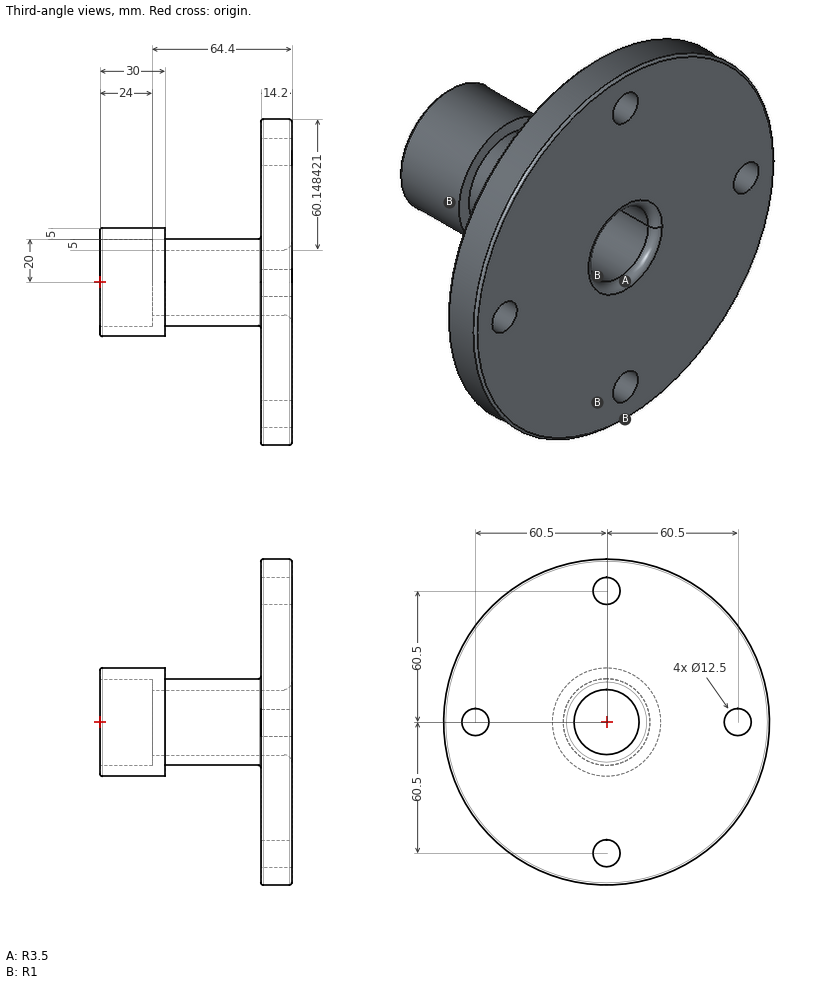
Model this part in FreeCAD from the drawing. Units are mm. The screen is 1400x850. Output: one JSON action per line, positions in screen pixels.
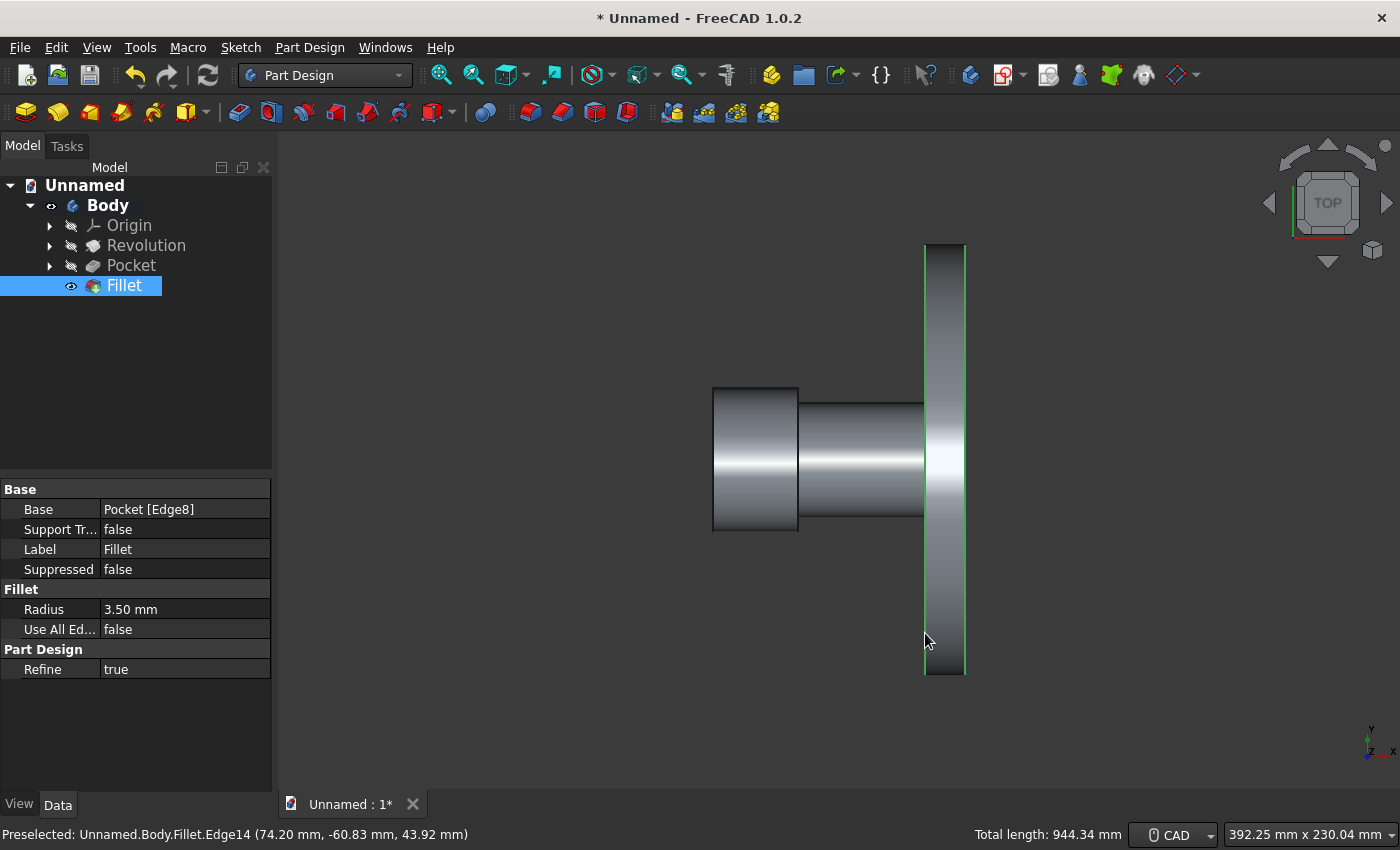
{"action": "left_click", "coordinate": [713, 517], "text": "ctrl"}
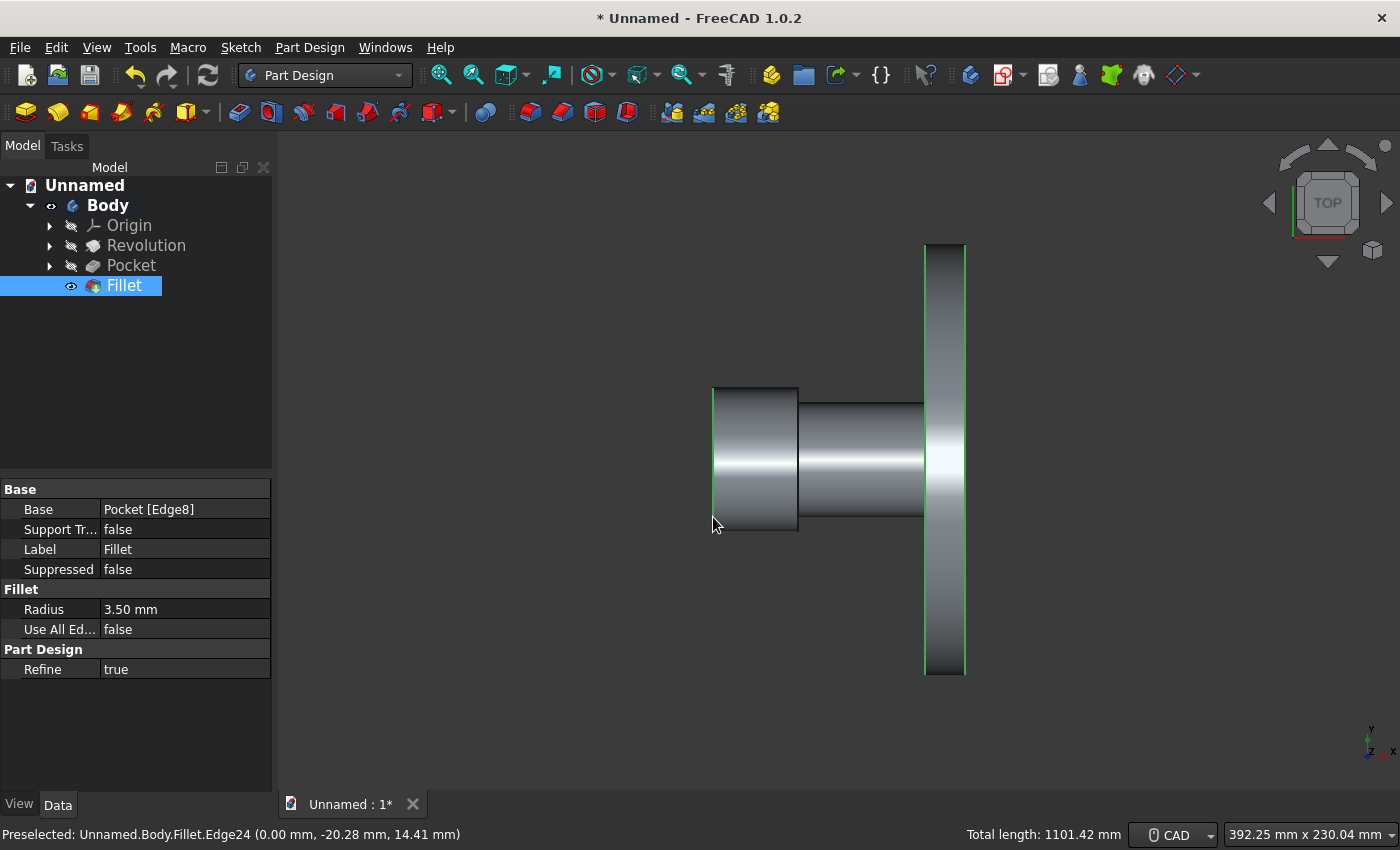
{"action": "key", "text": "0"}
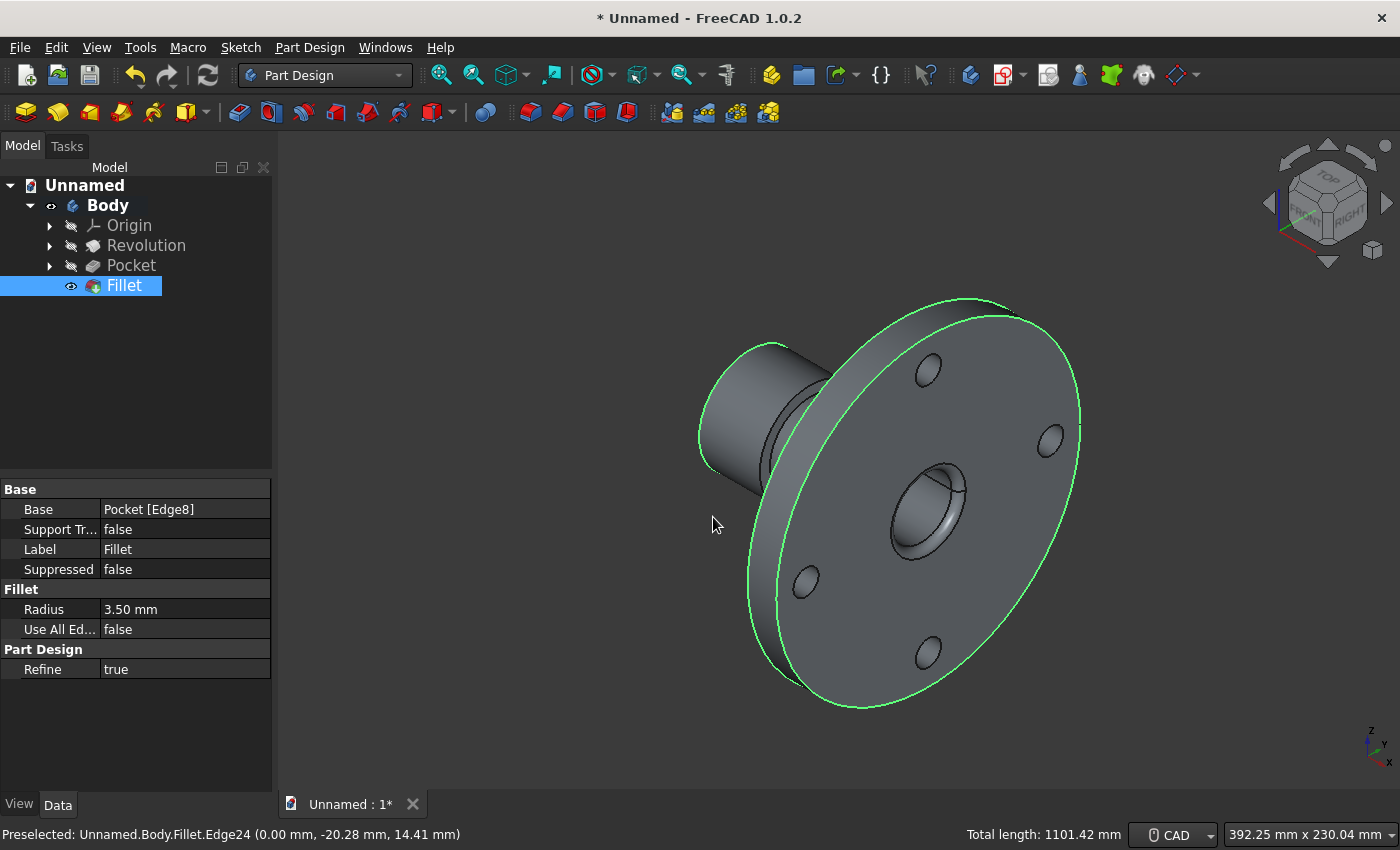
{"action": "key", "text": "1"}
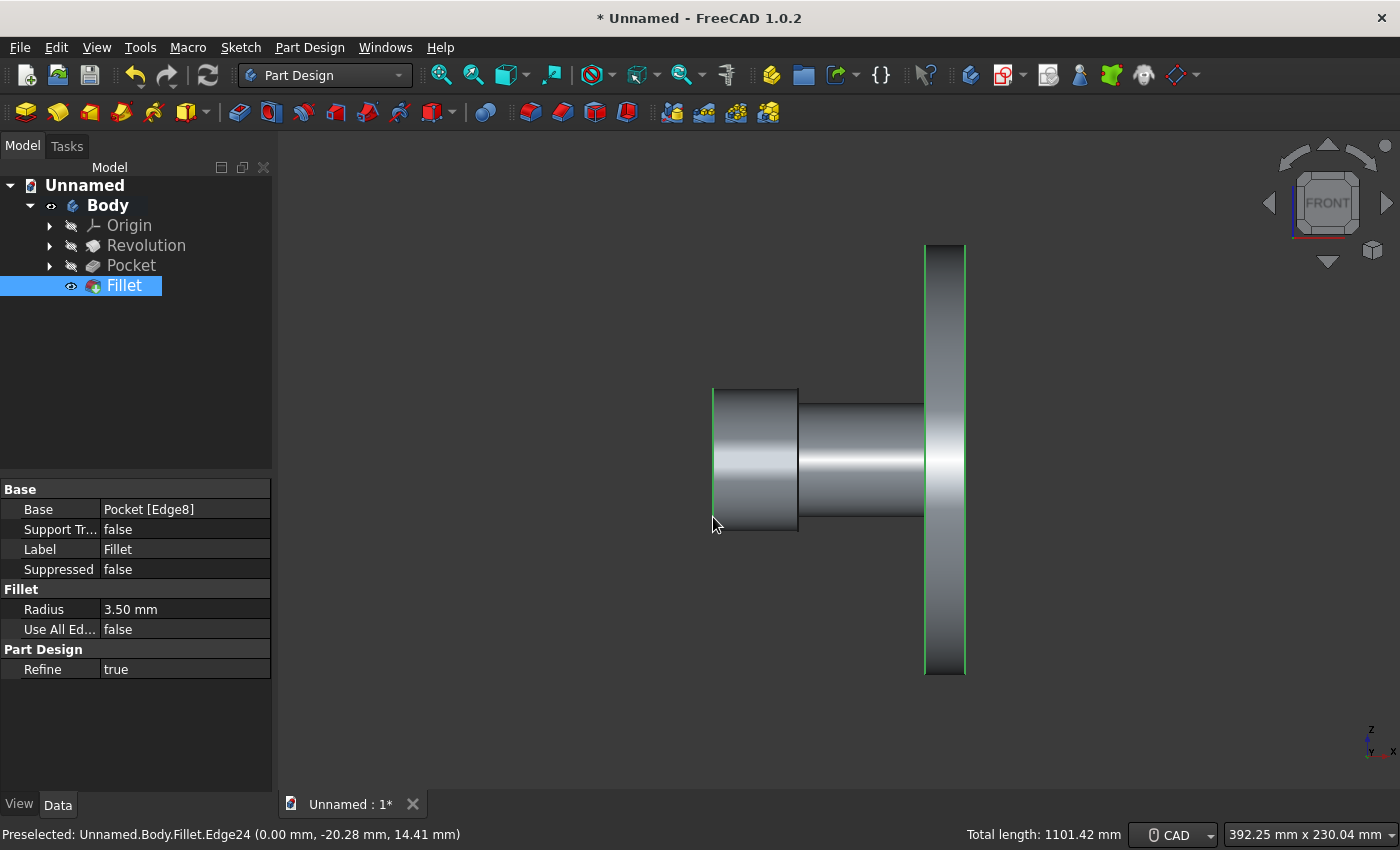
{"action": "key", "text": "3"}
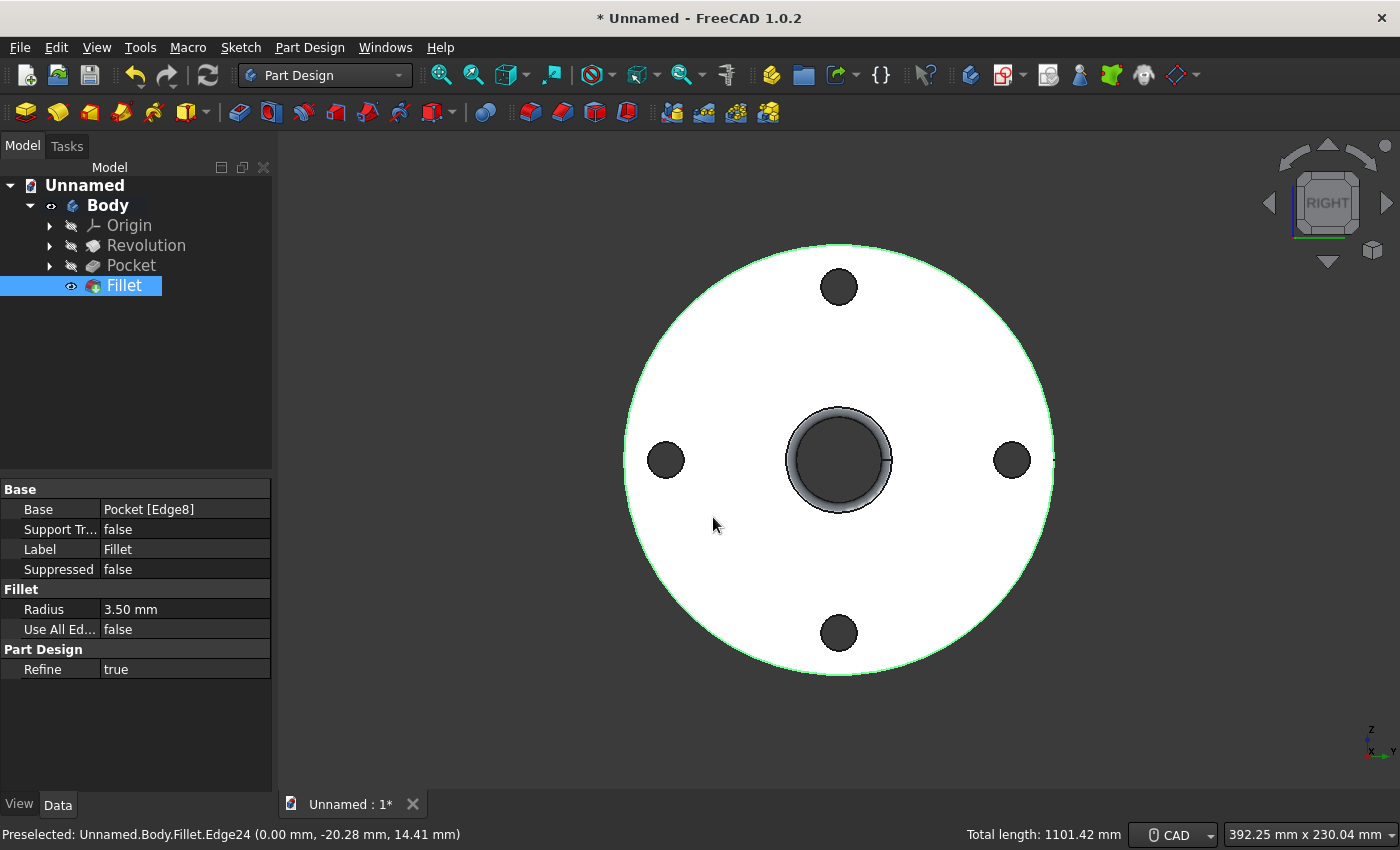
{"action": "key", "text": "5"}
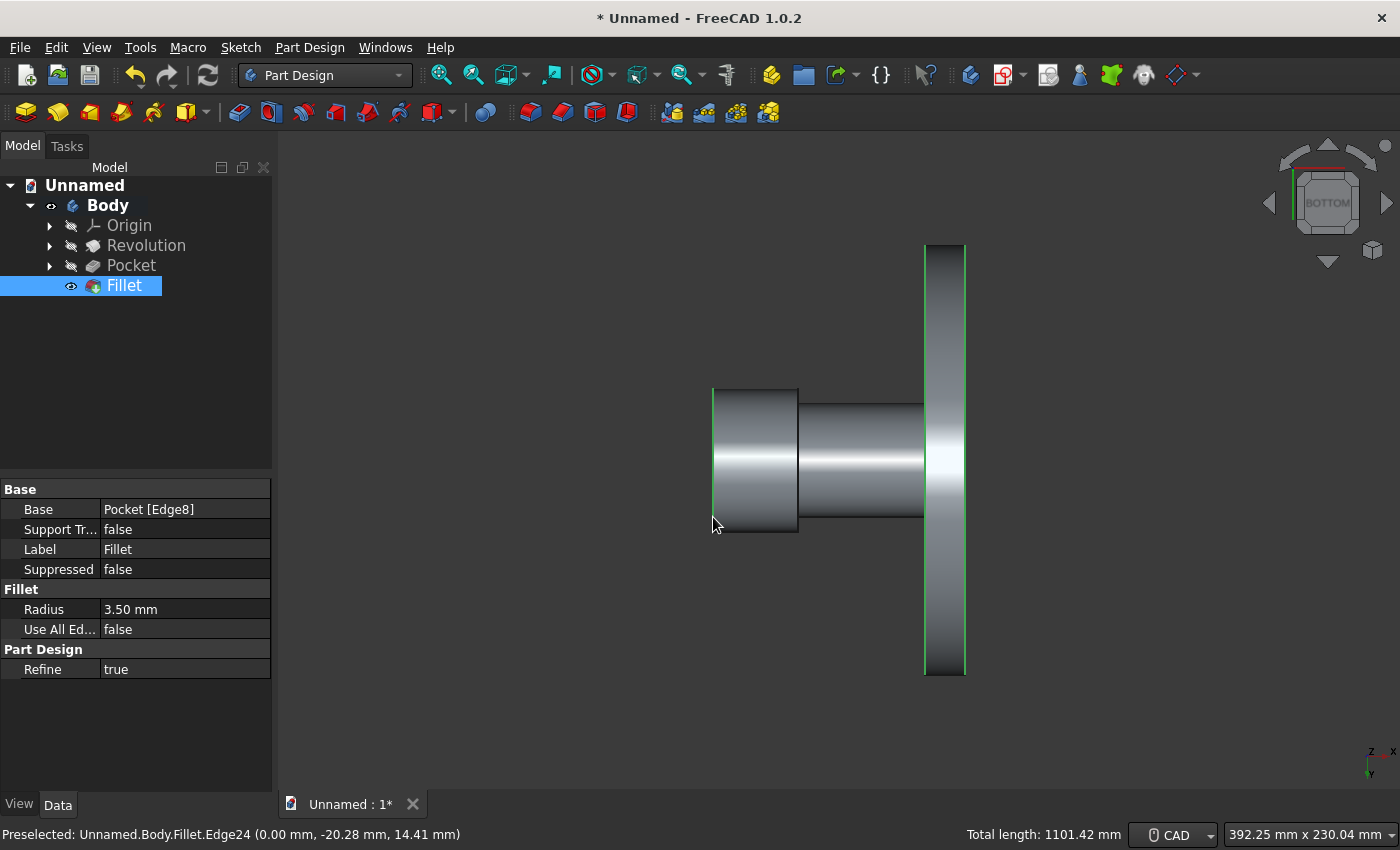
{"action": "key", "text": "4"}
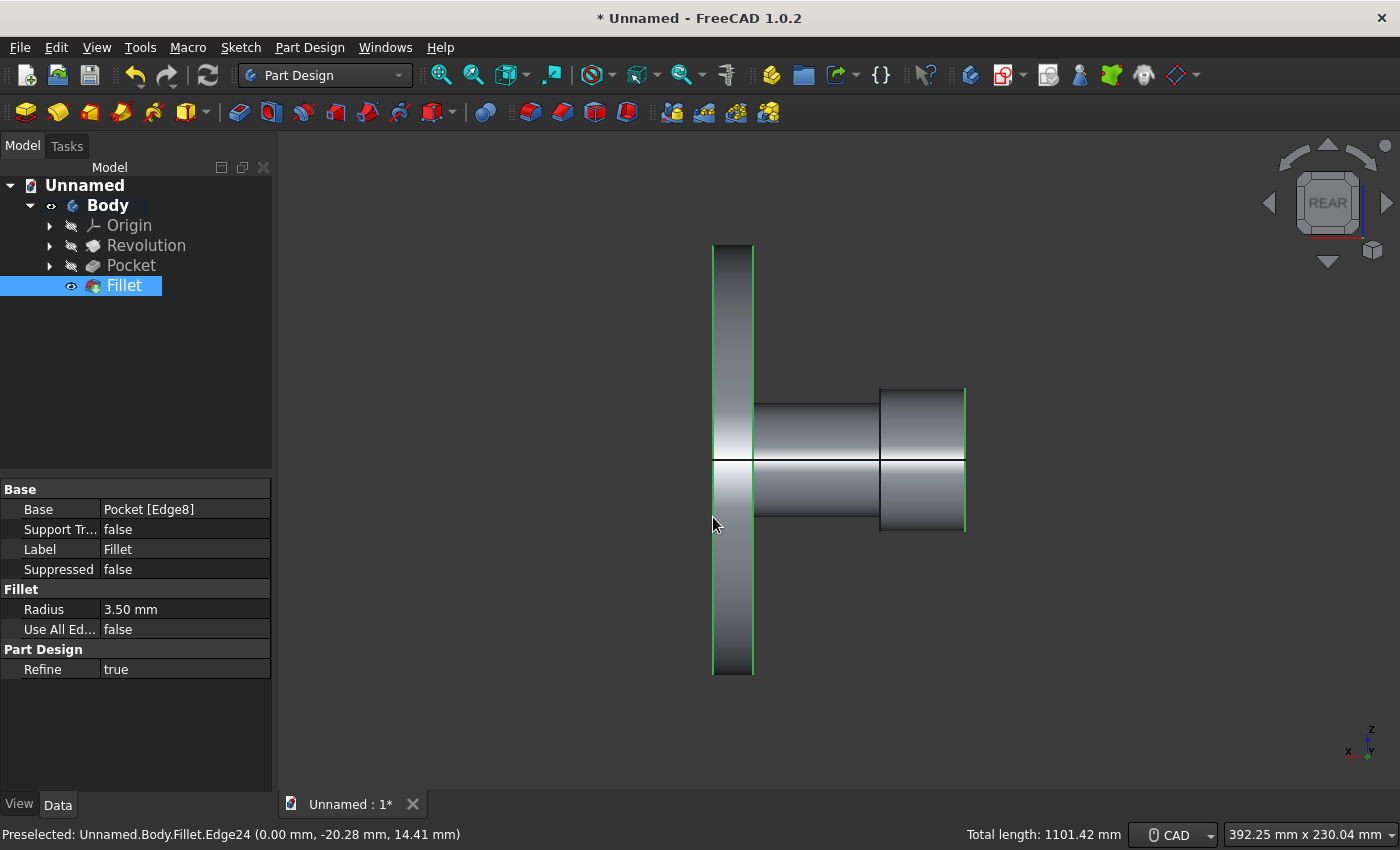
{"action": "key", "text": "6"}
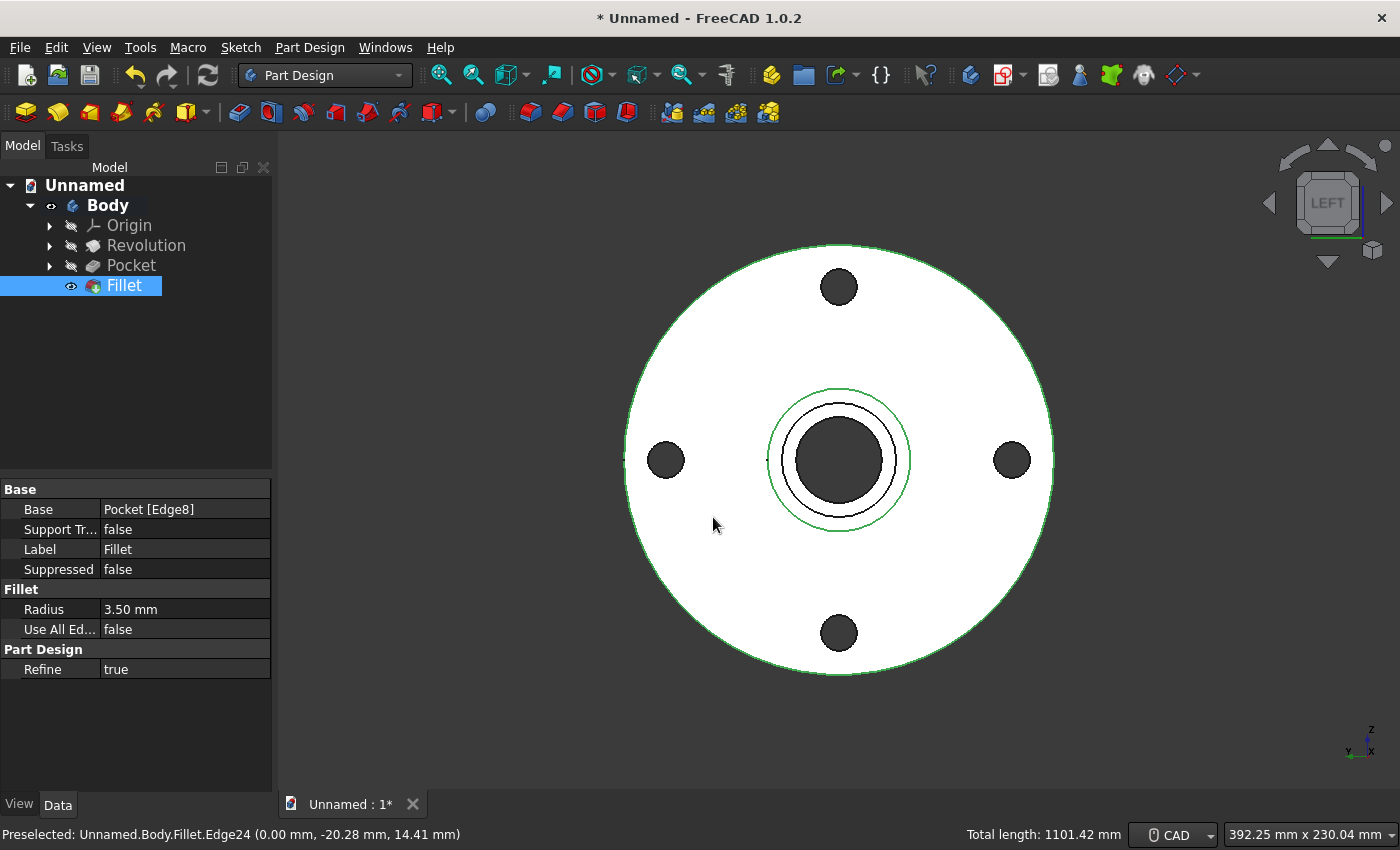
{"action": "key", "text": "v 3"}